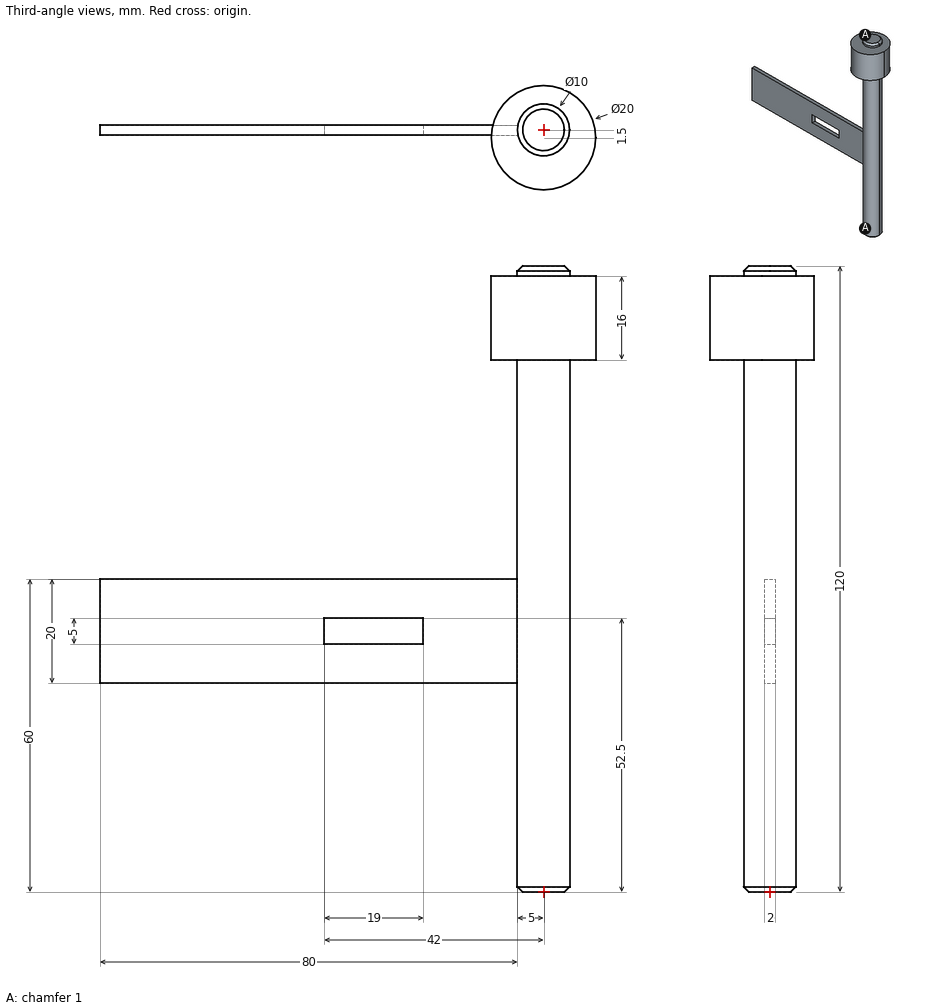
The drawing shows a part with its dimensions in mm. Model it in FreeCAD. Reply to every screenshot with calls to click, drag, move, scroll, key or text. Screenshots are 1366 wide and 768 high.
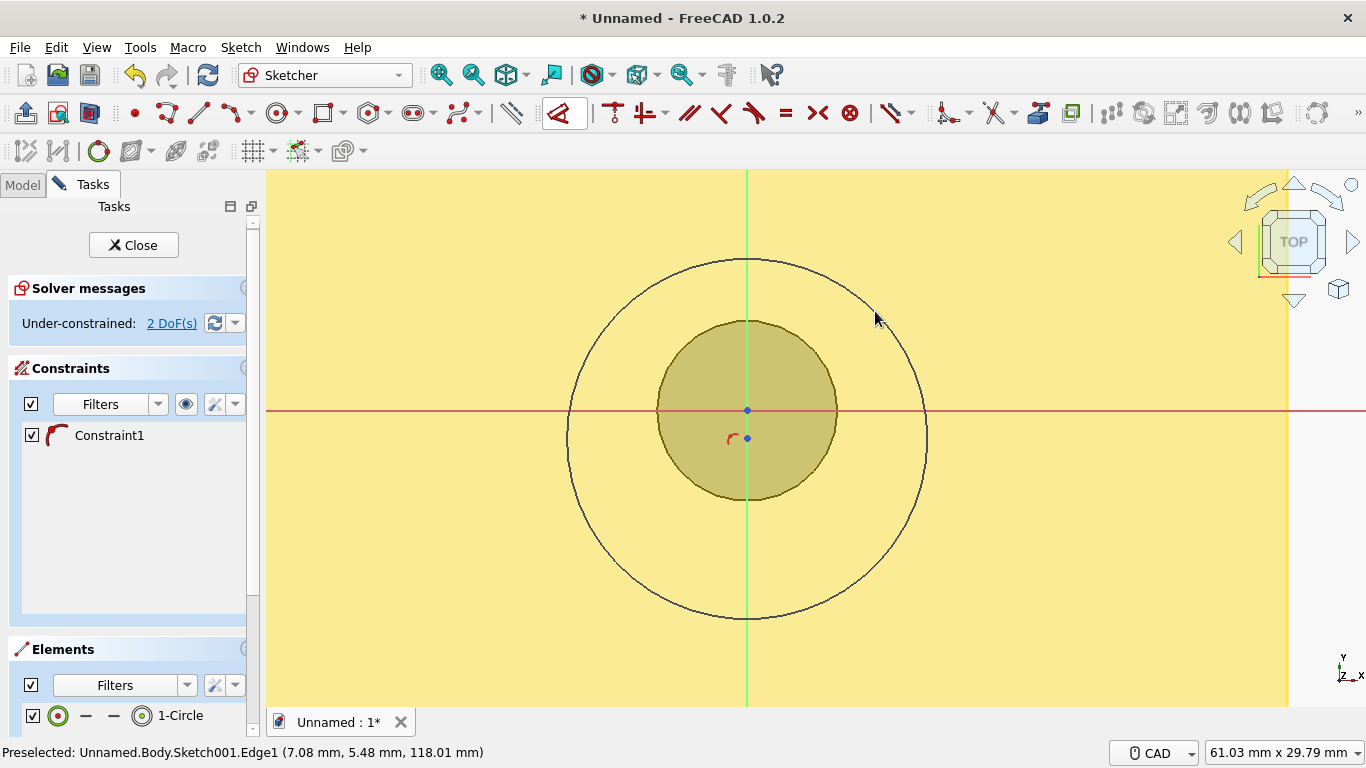
click(874, 311)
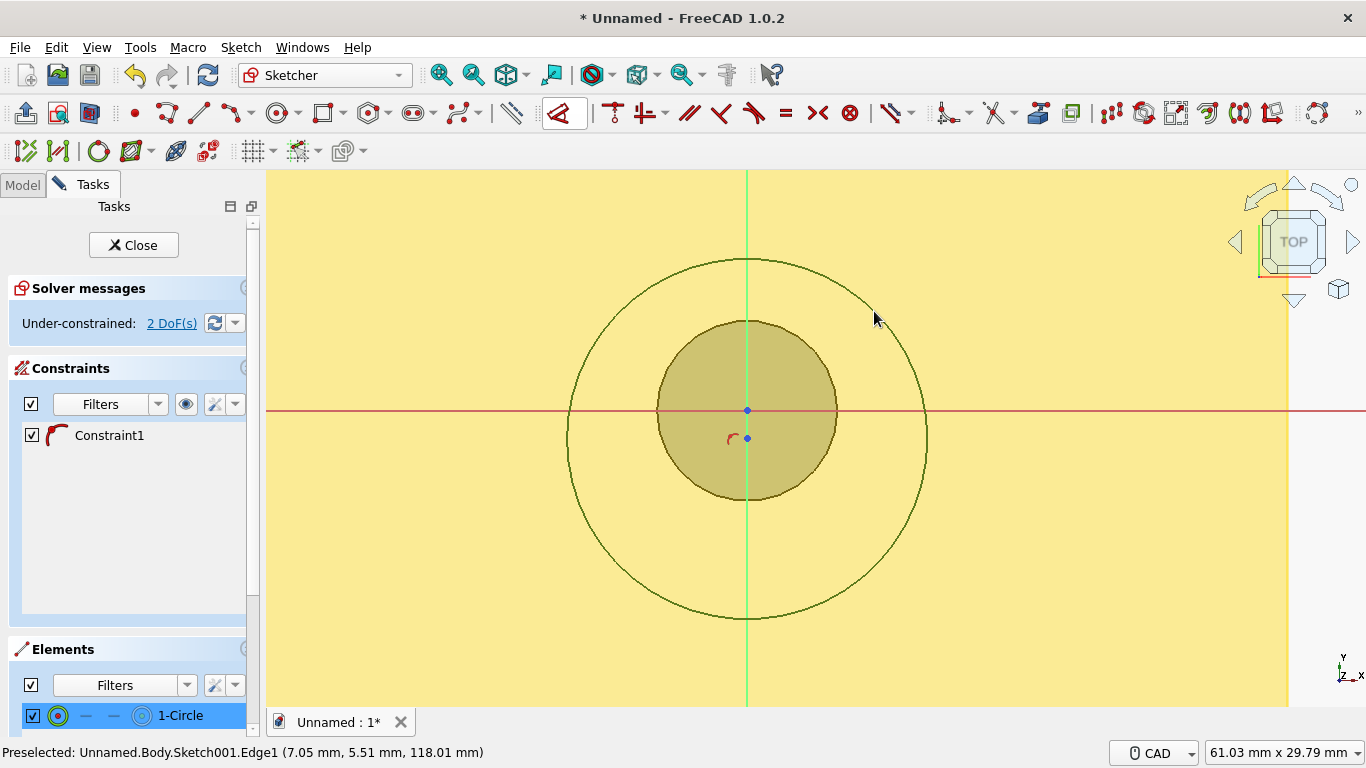
key(k)
key(o)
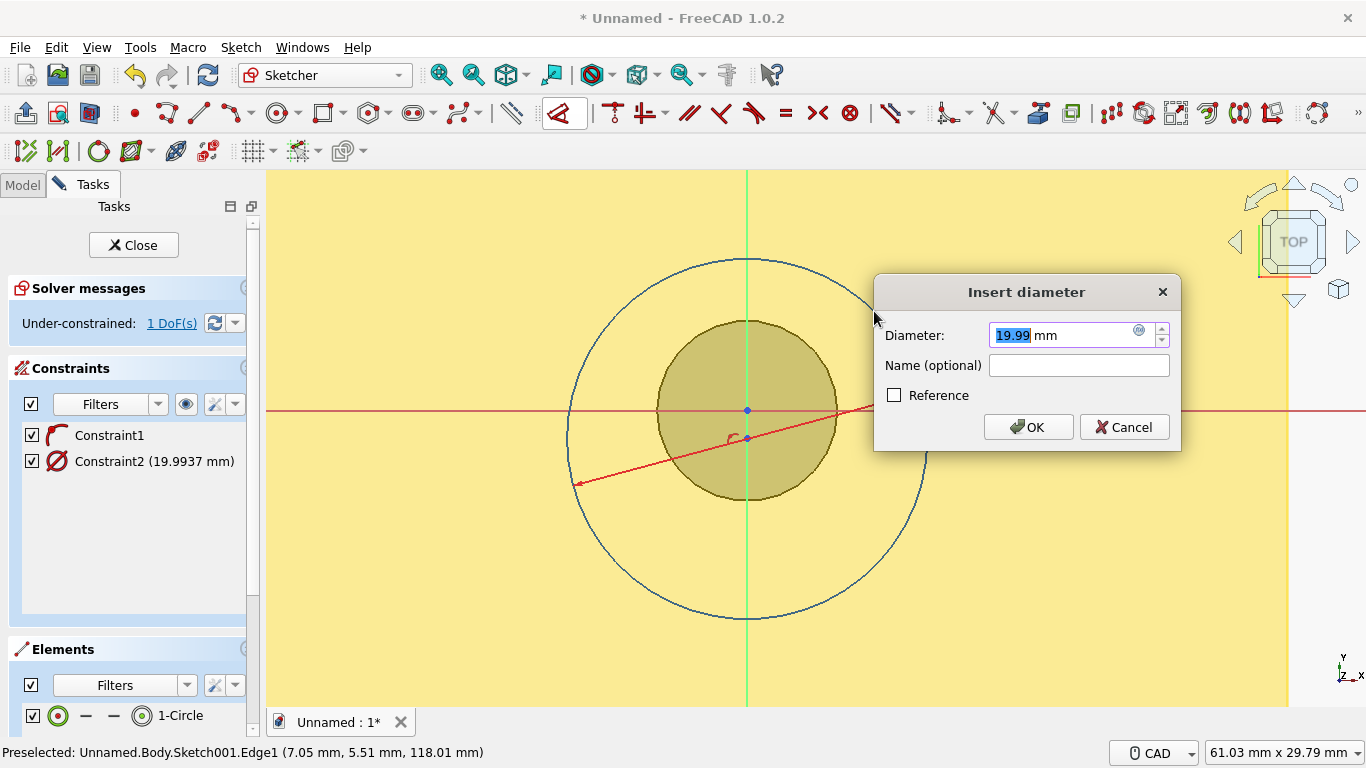
text(20)
key(Return)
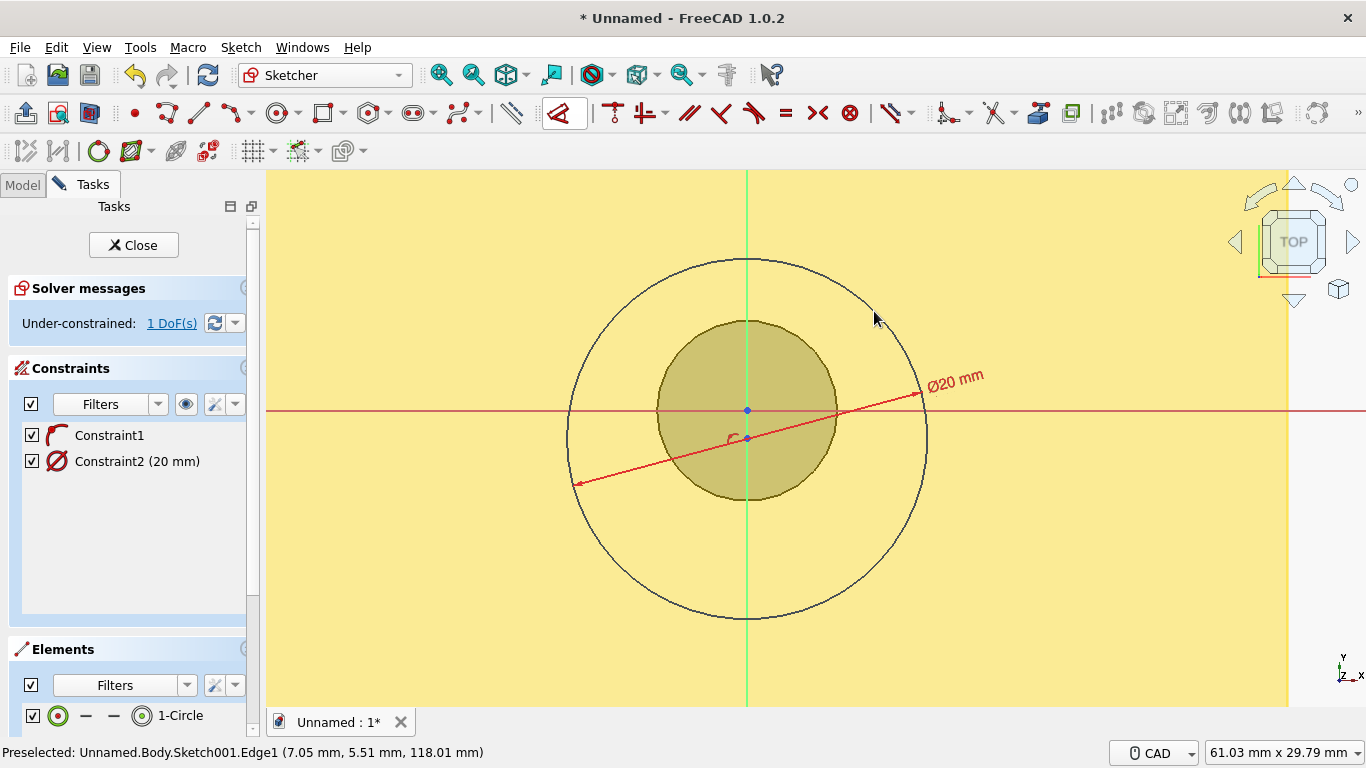
scroll(747, 439, up, 2)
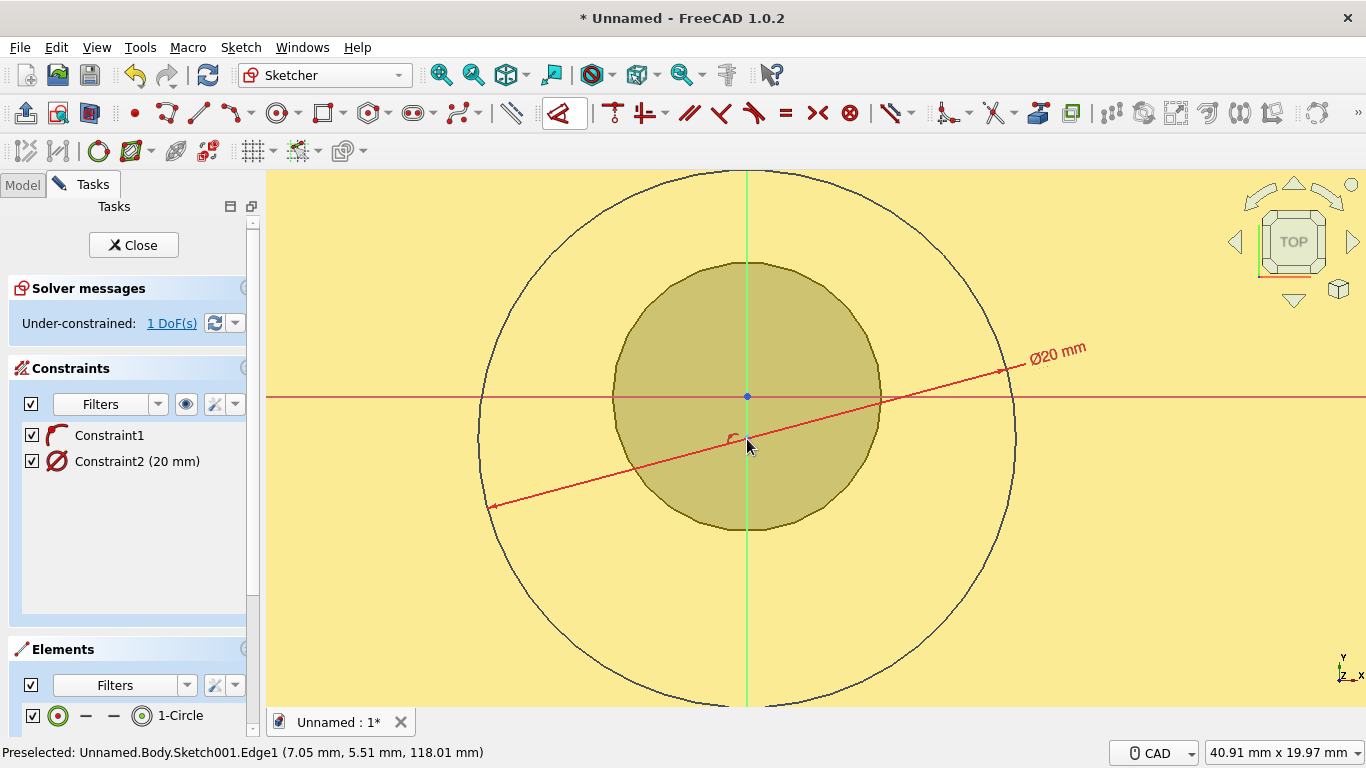
click(747, 439)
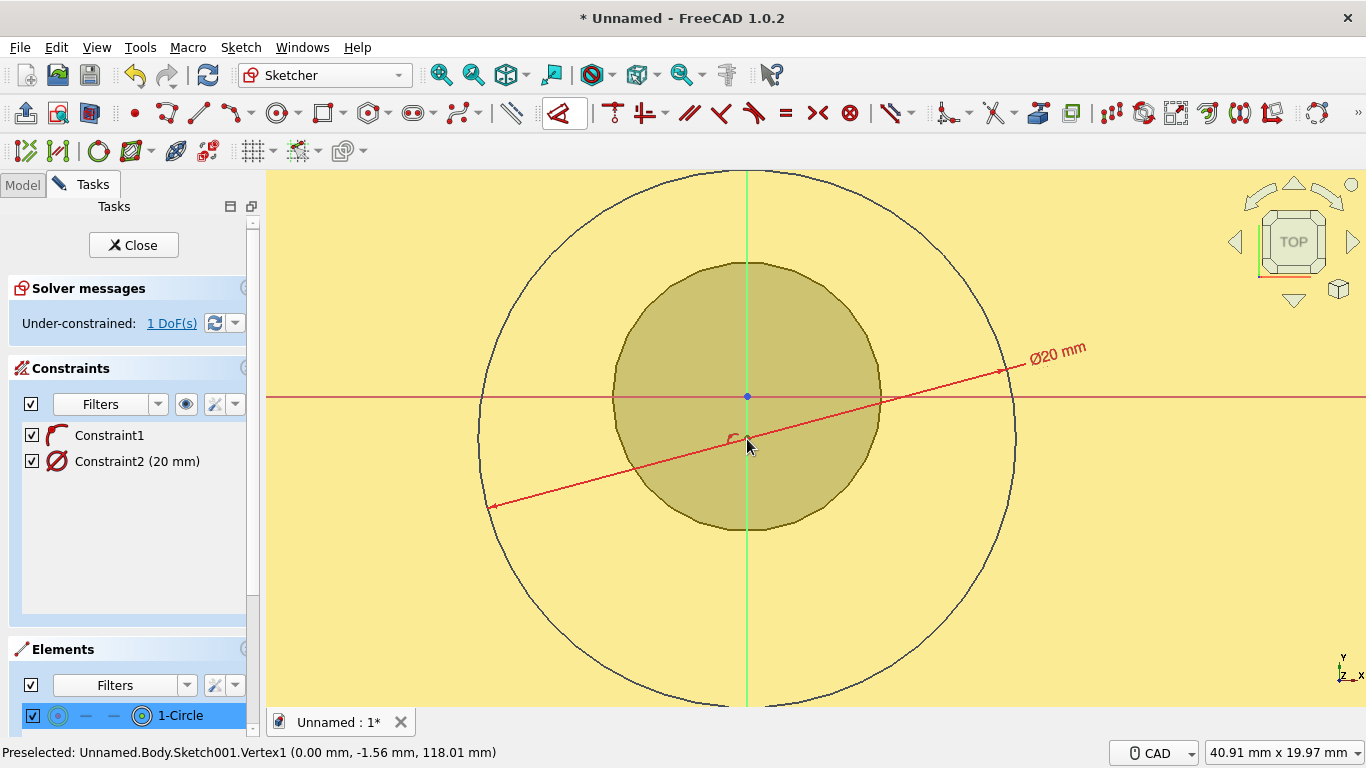
click(582, 114)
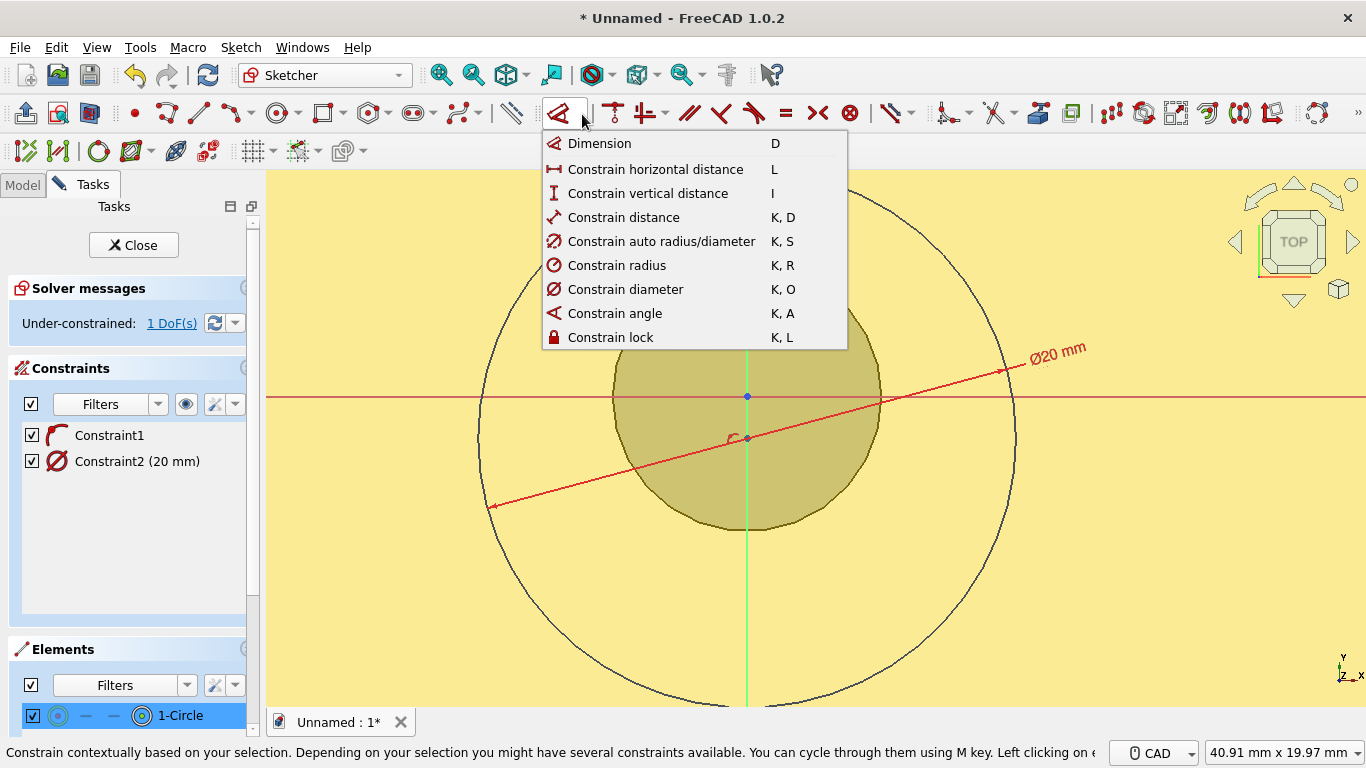
click(695, 193)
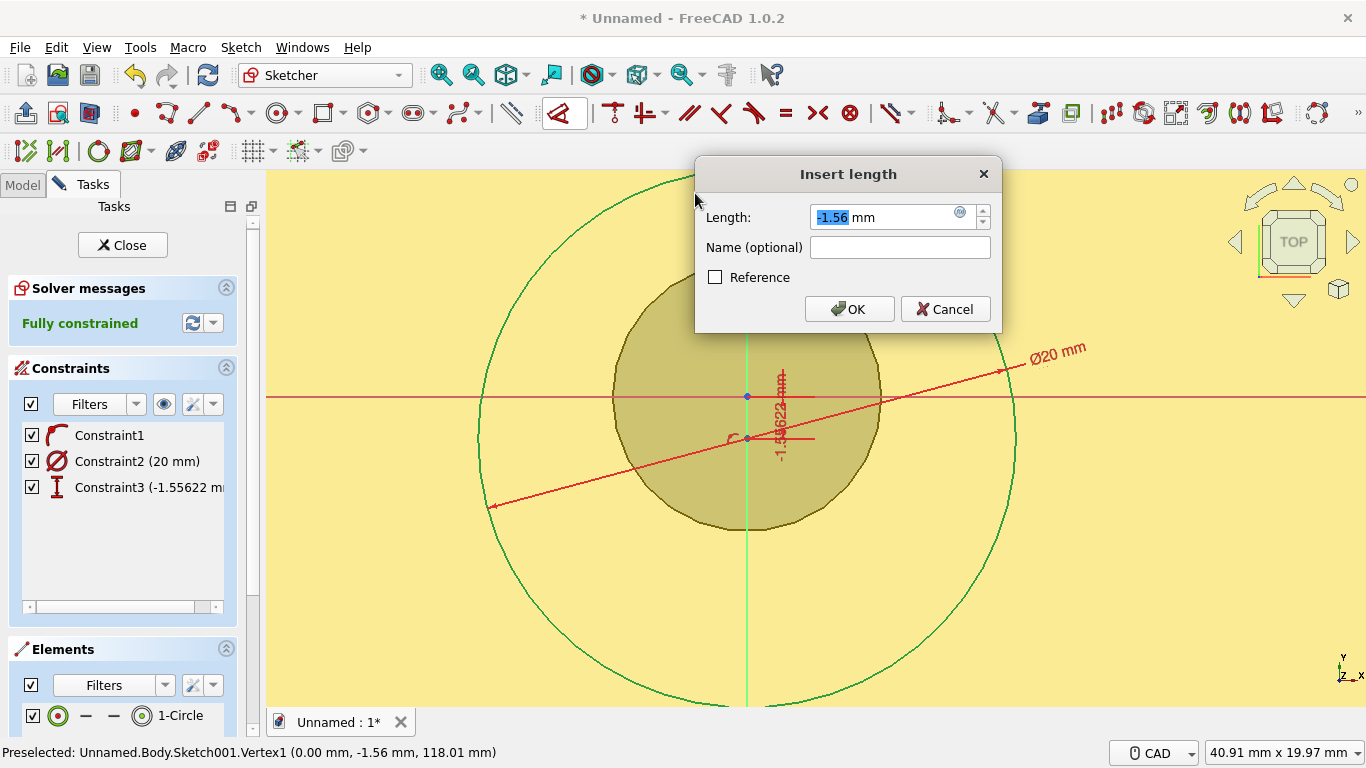
text(-1.5)
key(Return)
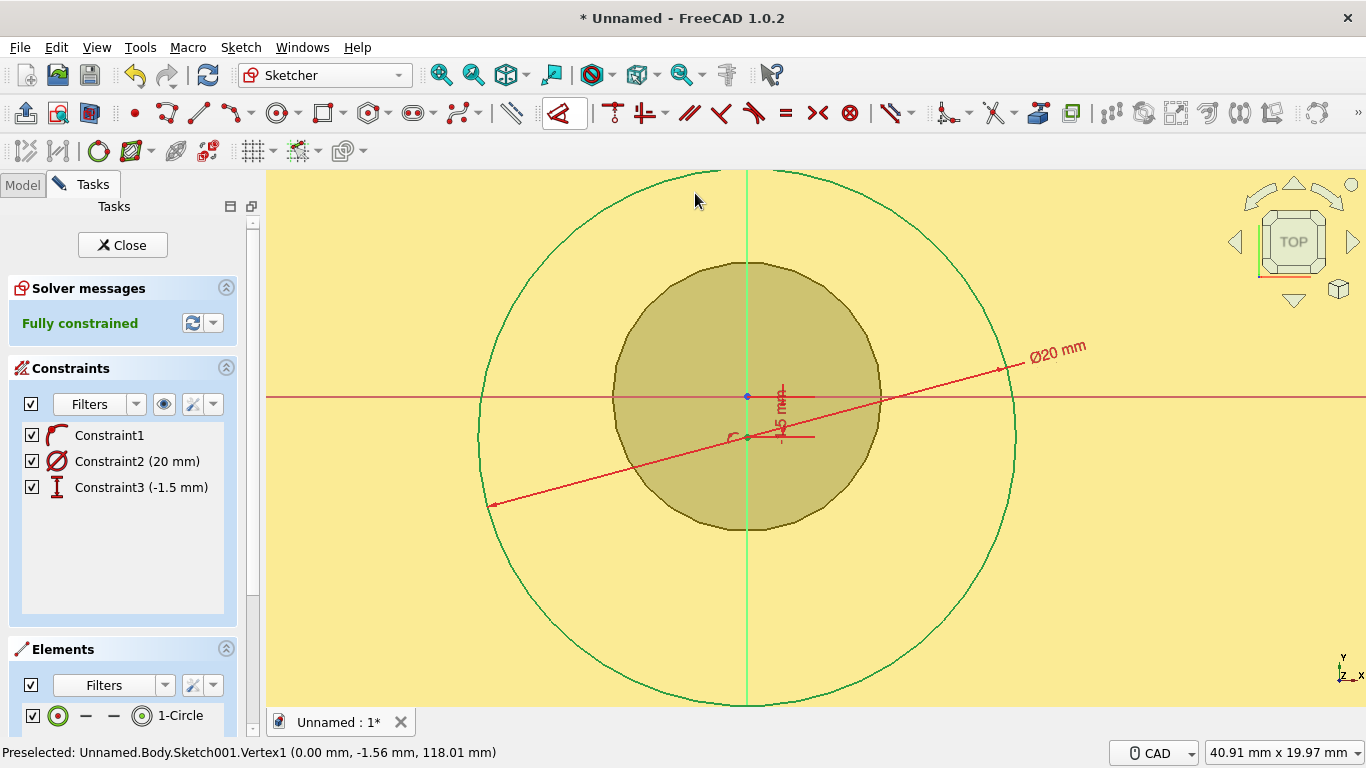
click(123, 245)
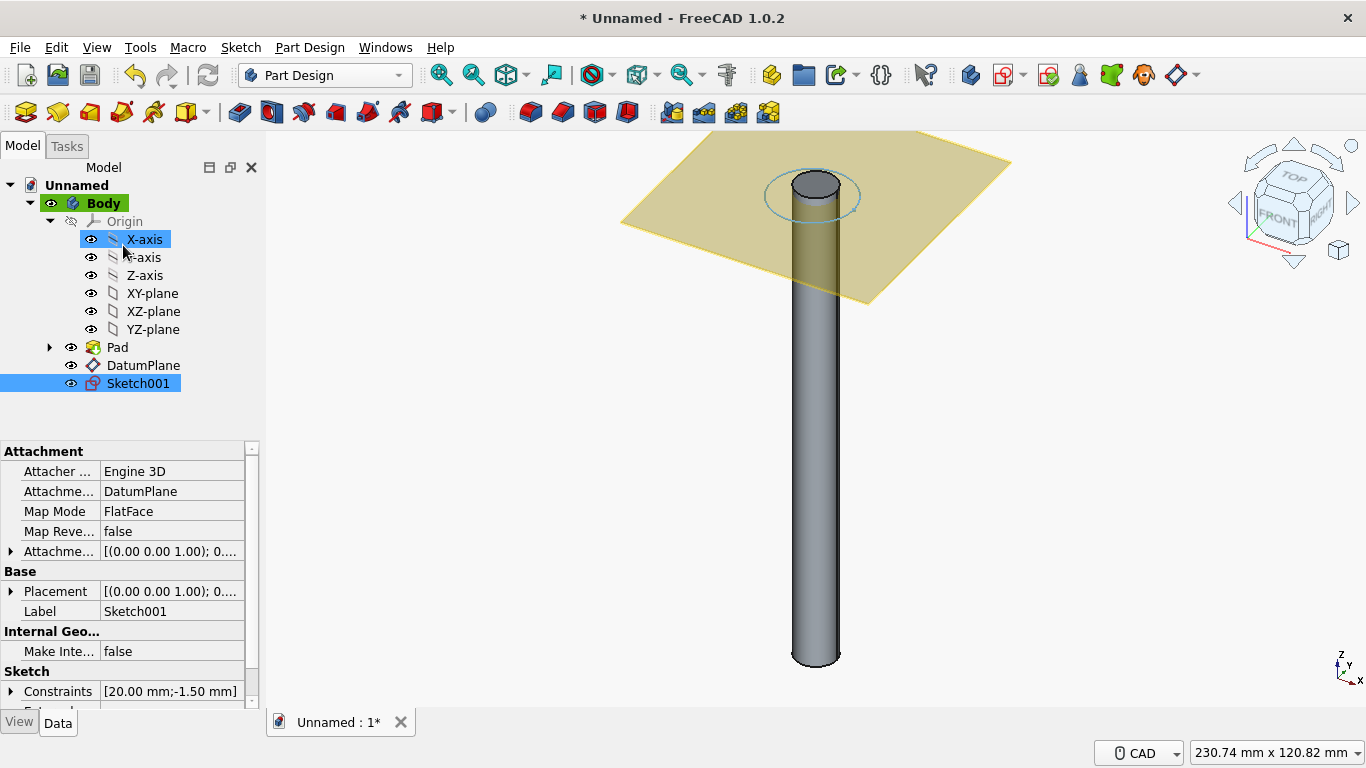
click(26, 112)